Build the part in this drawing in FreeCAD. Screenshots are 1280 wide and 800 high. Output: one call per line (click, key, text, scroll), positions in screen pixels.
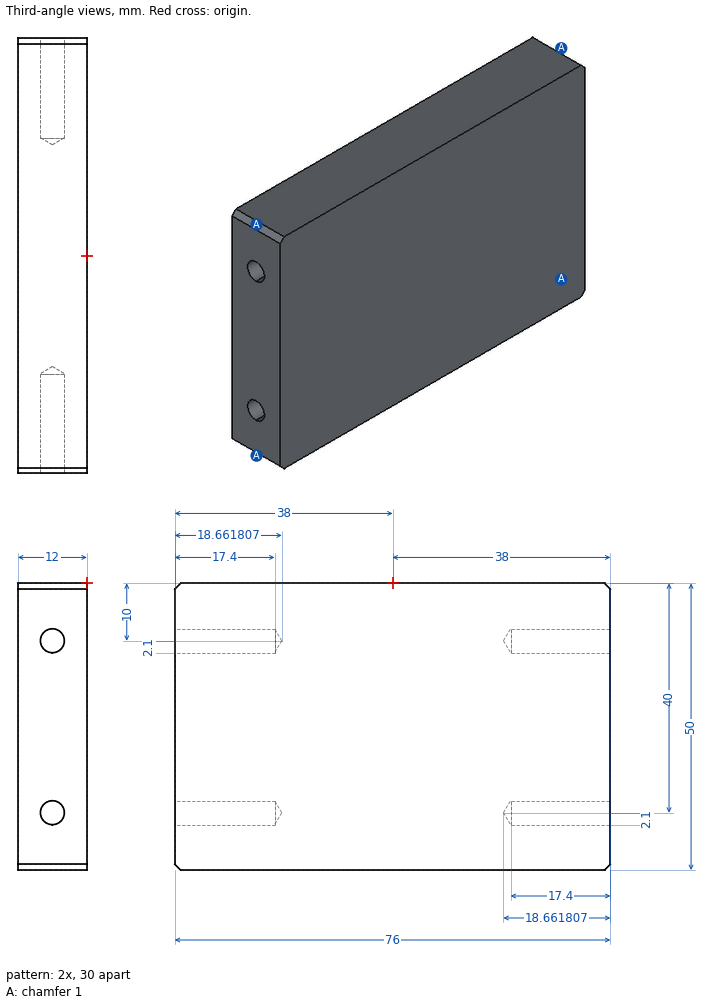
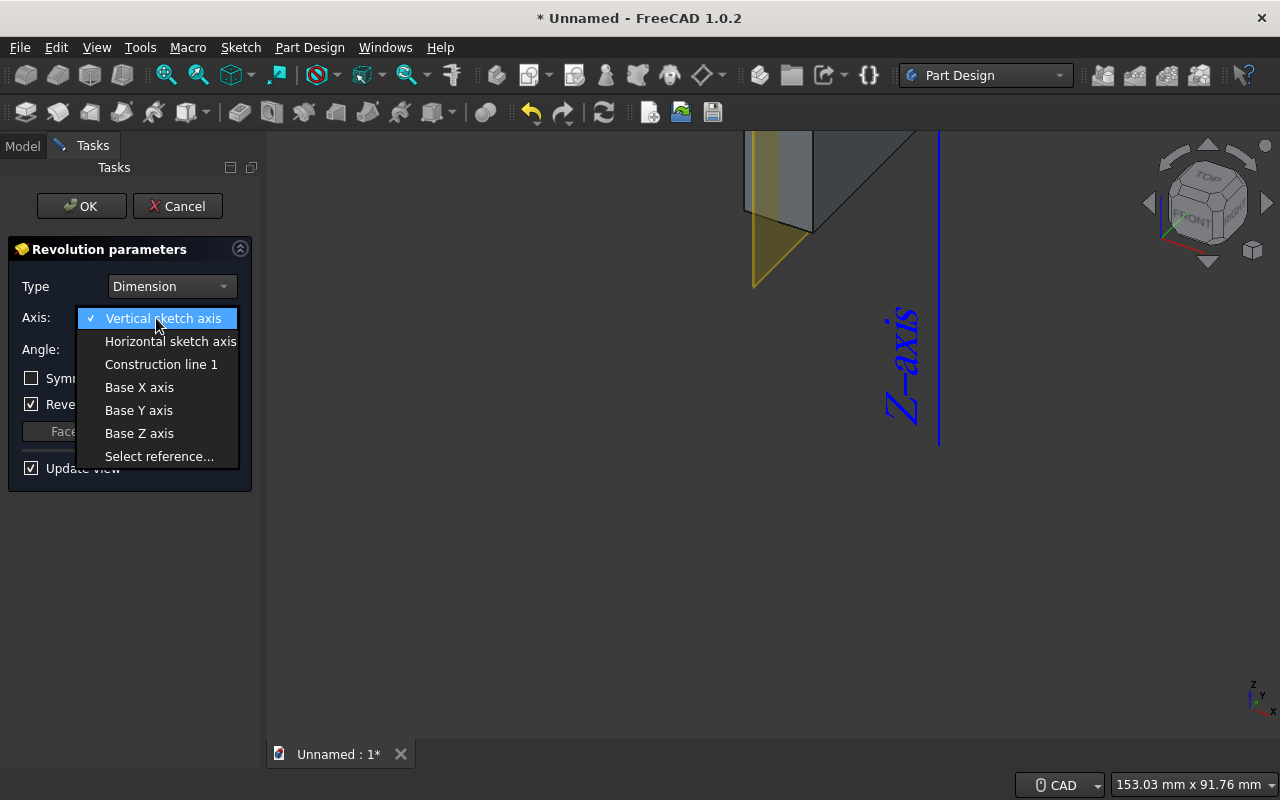
click(156, 364)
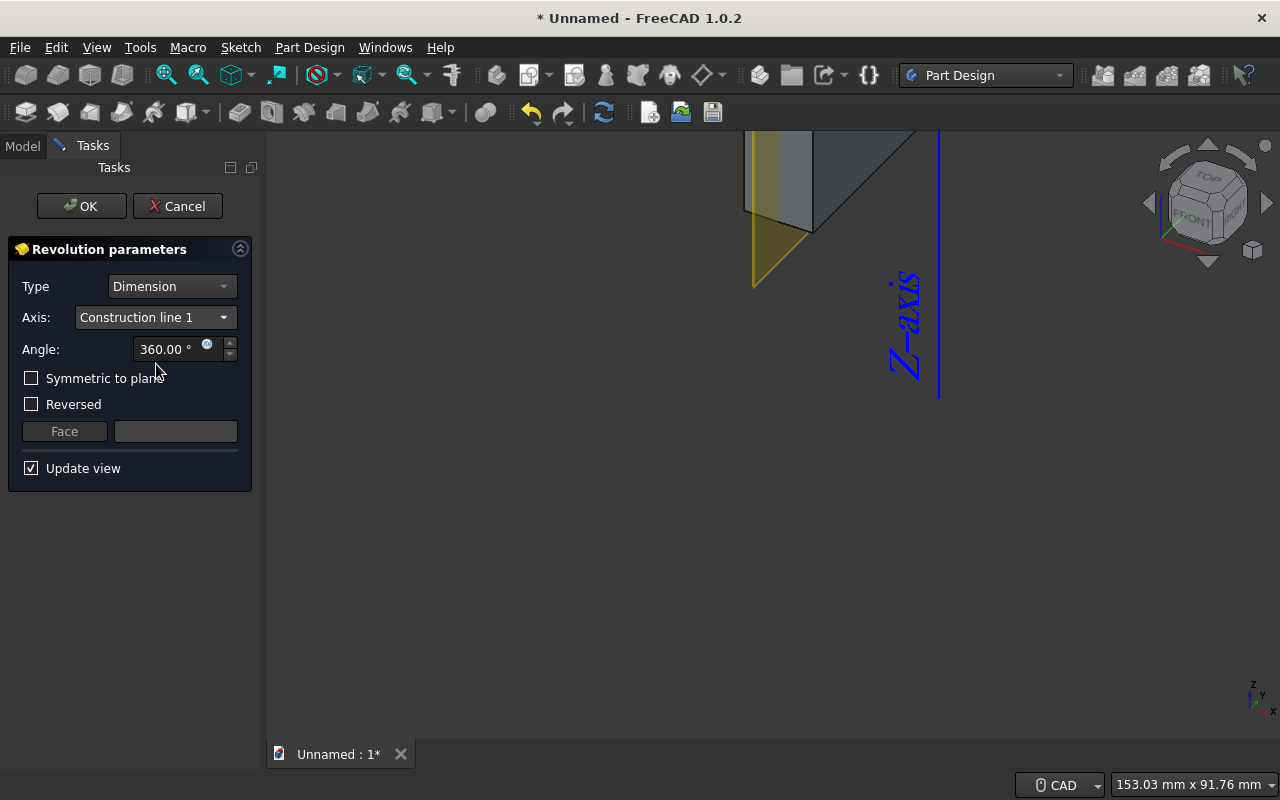
click(82, 206)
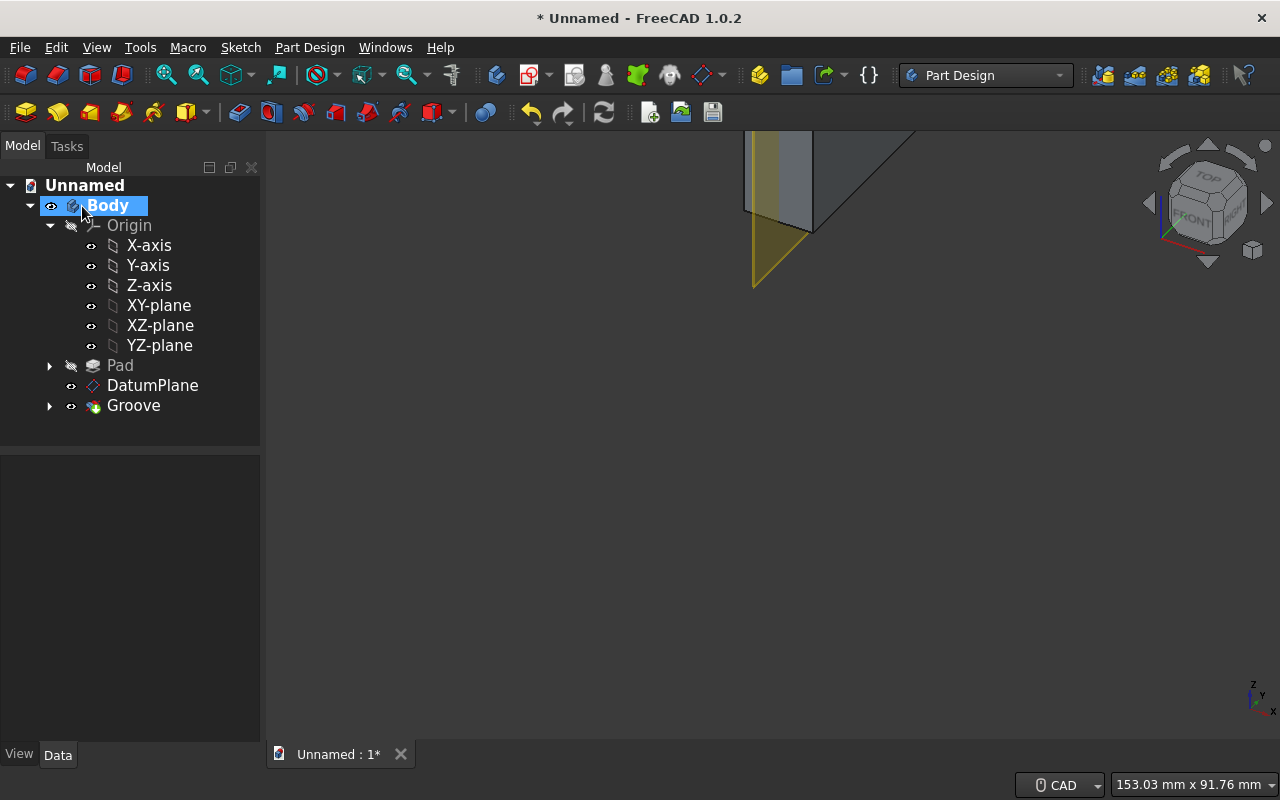
click(116, 386)
key(space)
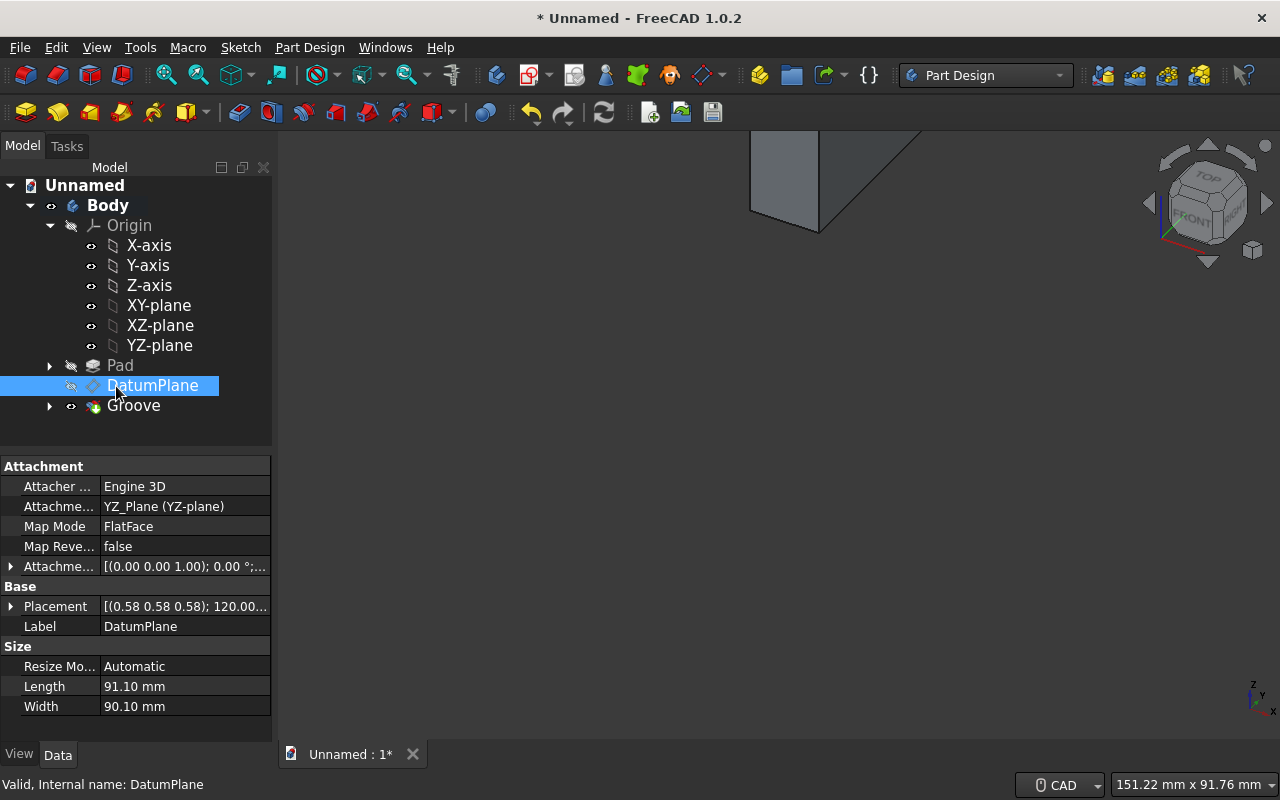
click(168, 76)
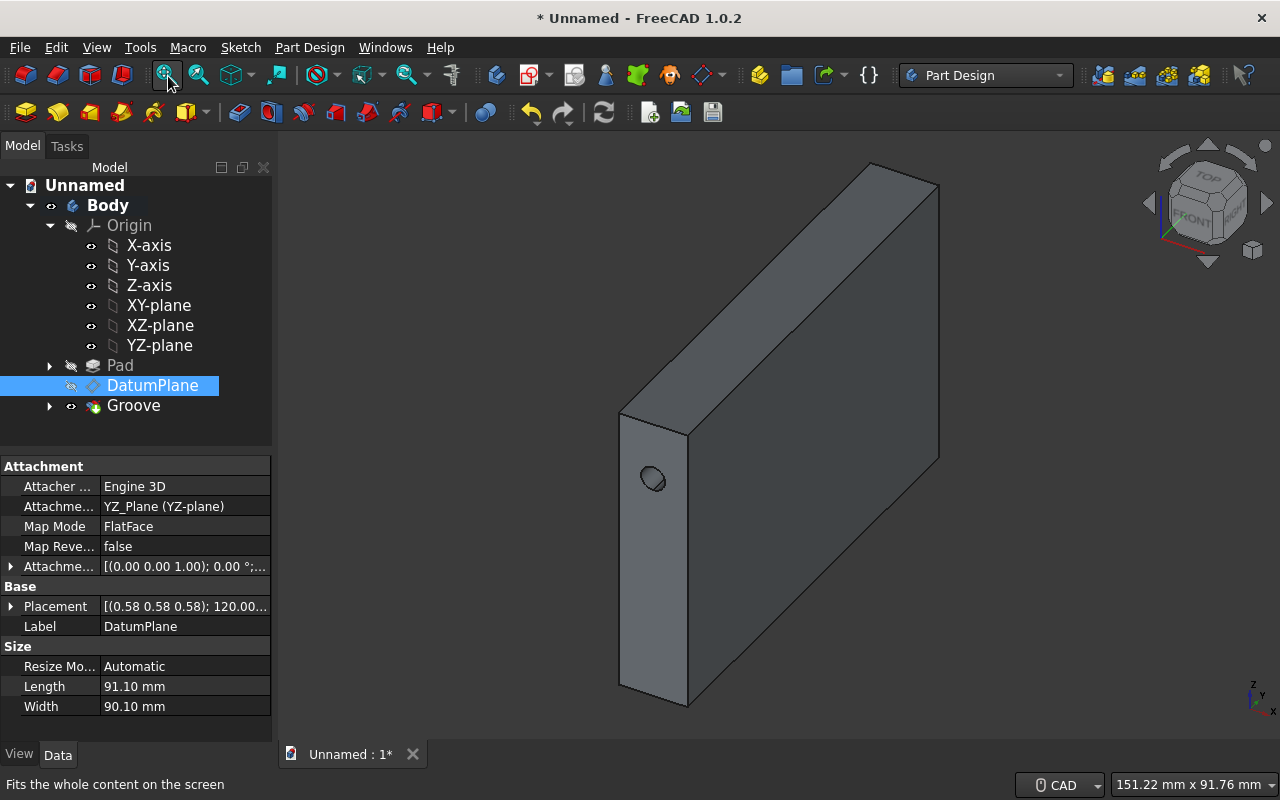
click(116, 406)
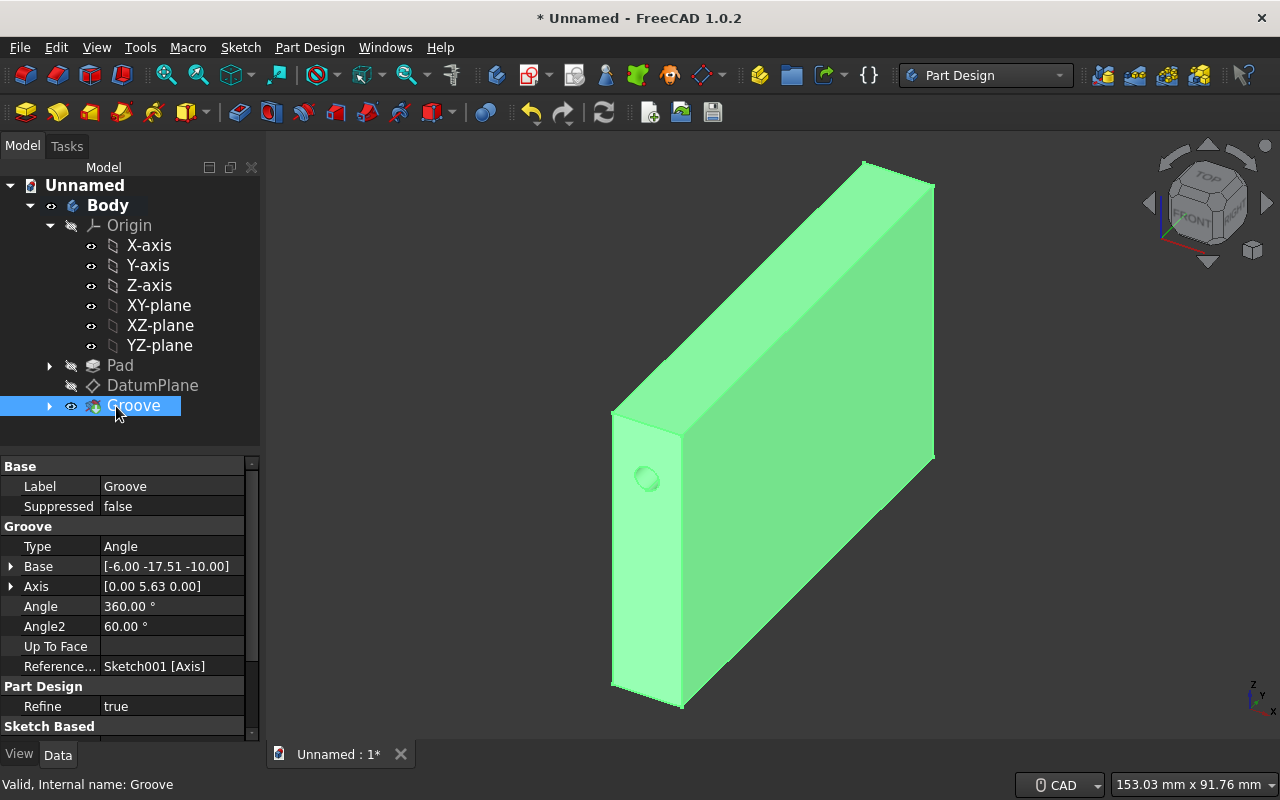
click(1136, 76)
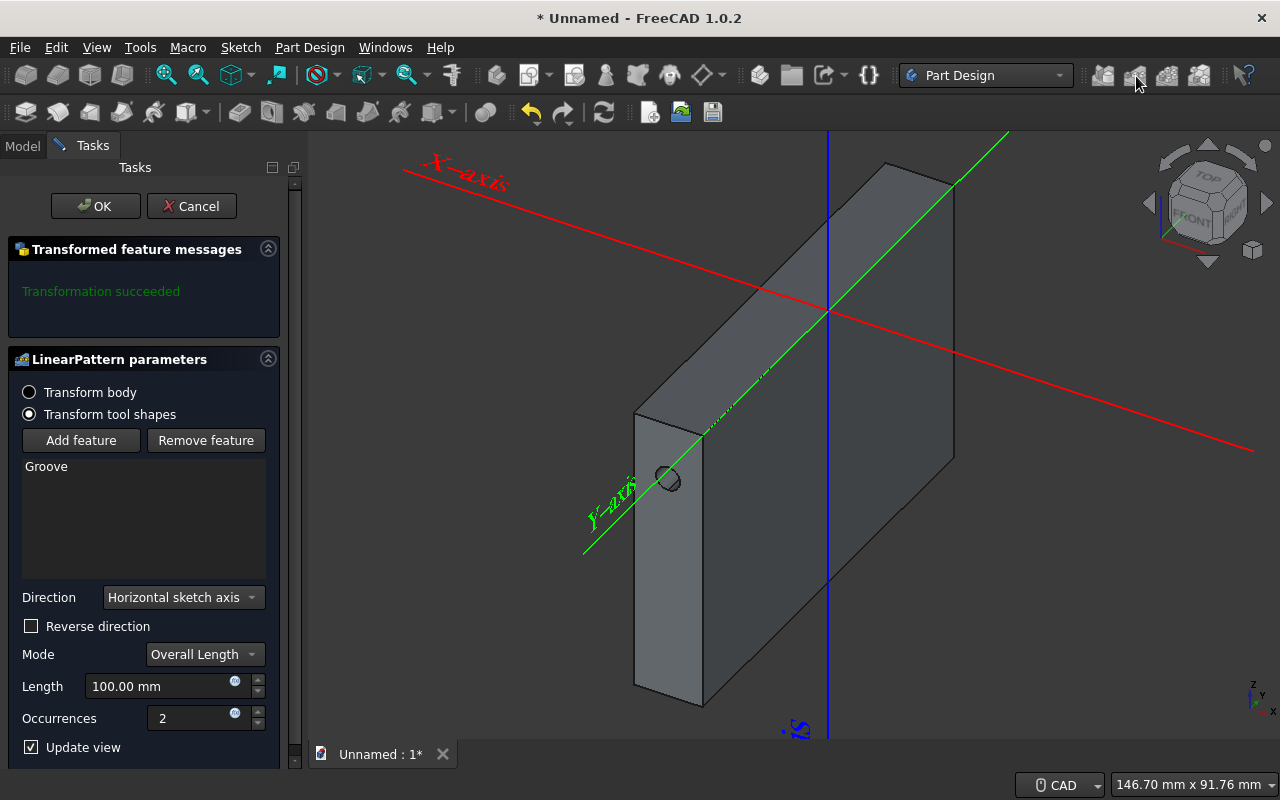
click(184, 598)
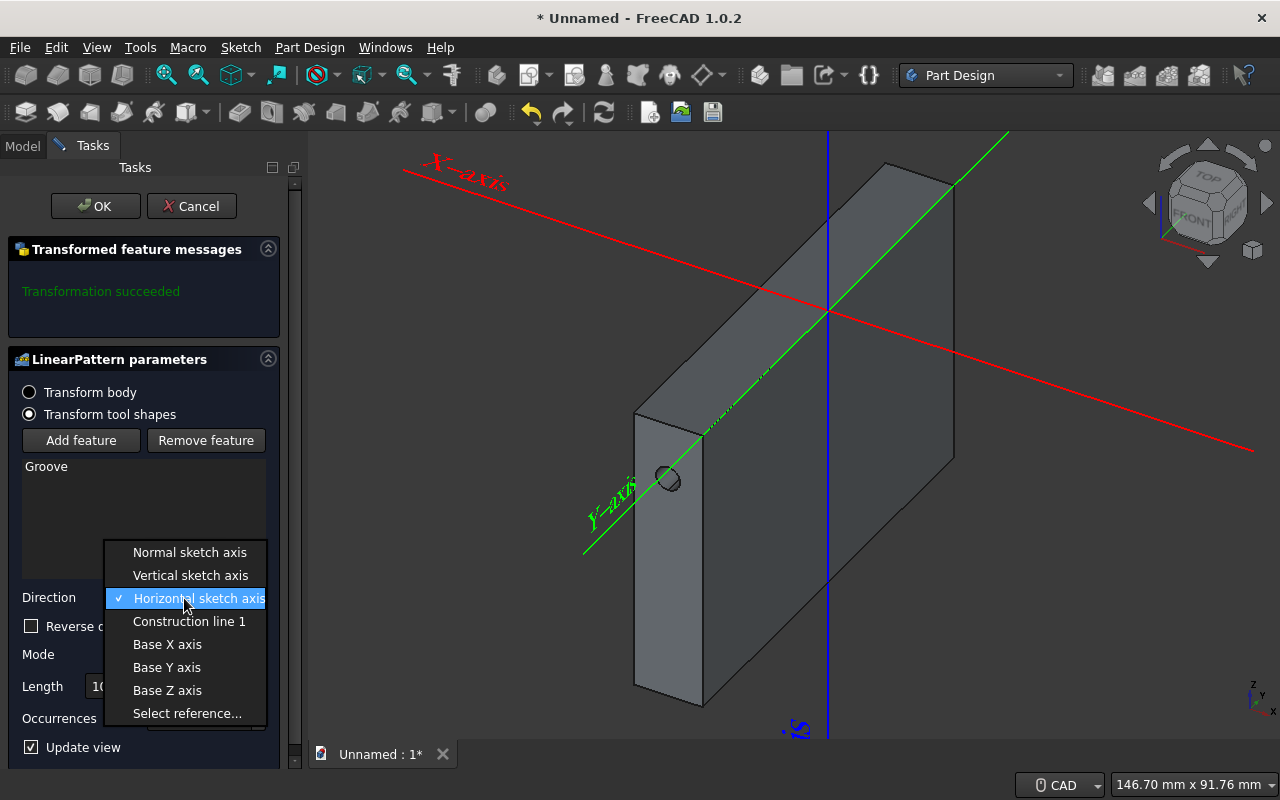
click(184, 690)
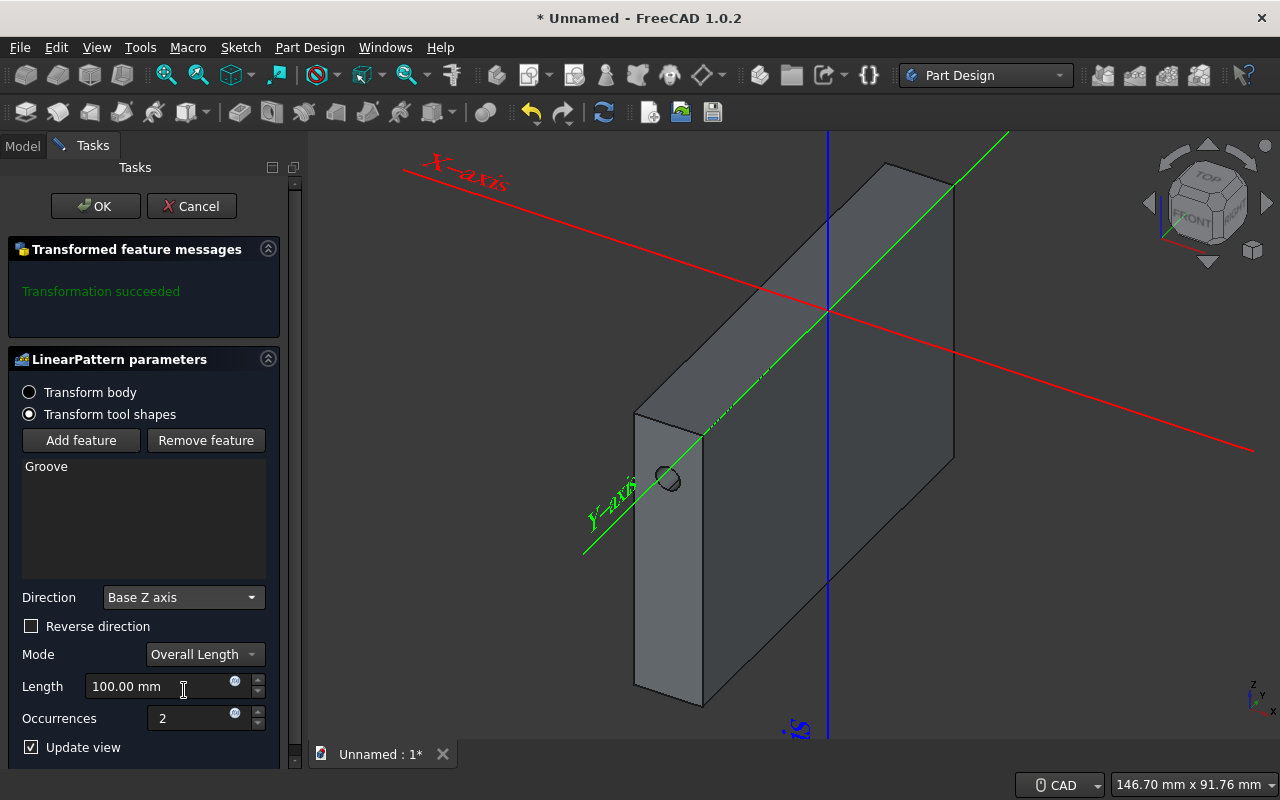
click(206, 654)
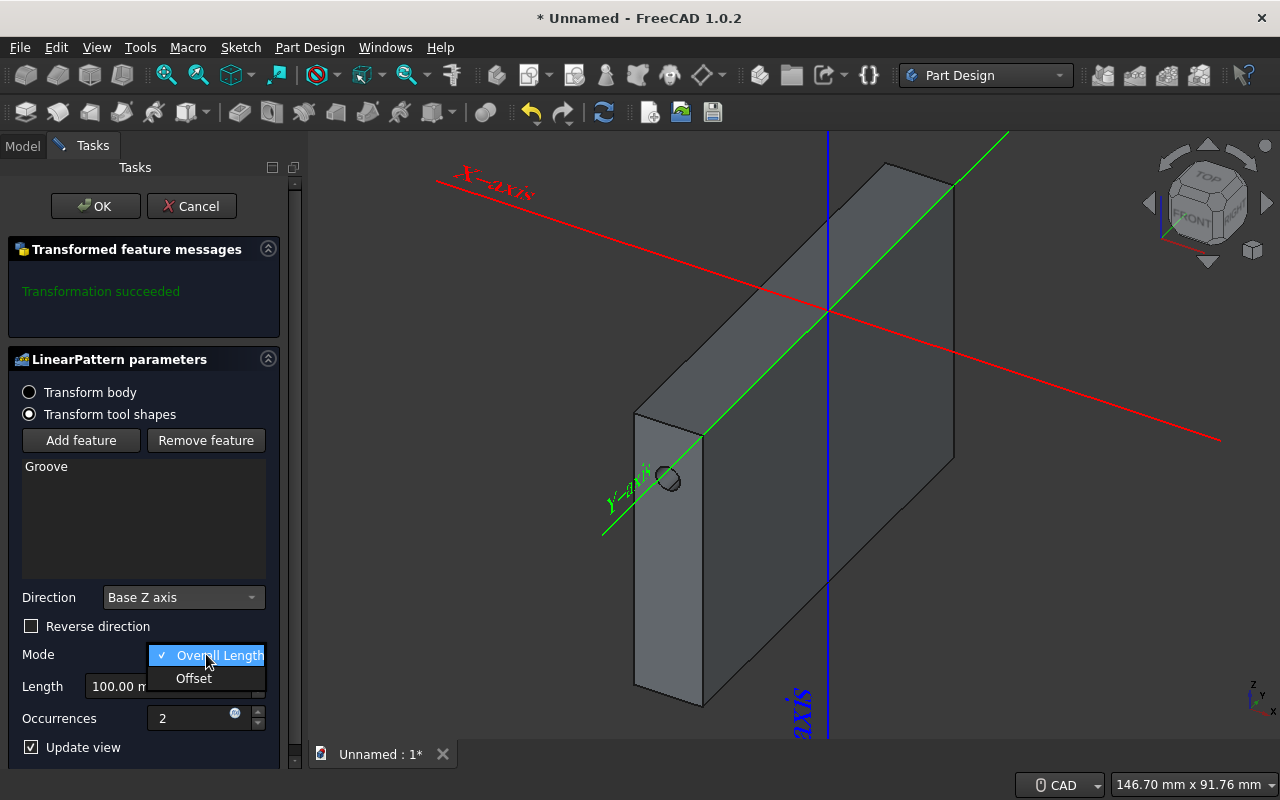
click(206, 678)